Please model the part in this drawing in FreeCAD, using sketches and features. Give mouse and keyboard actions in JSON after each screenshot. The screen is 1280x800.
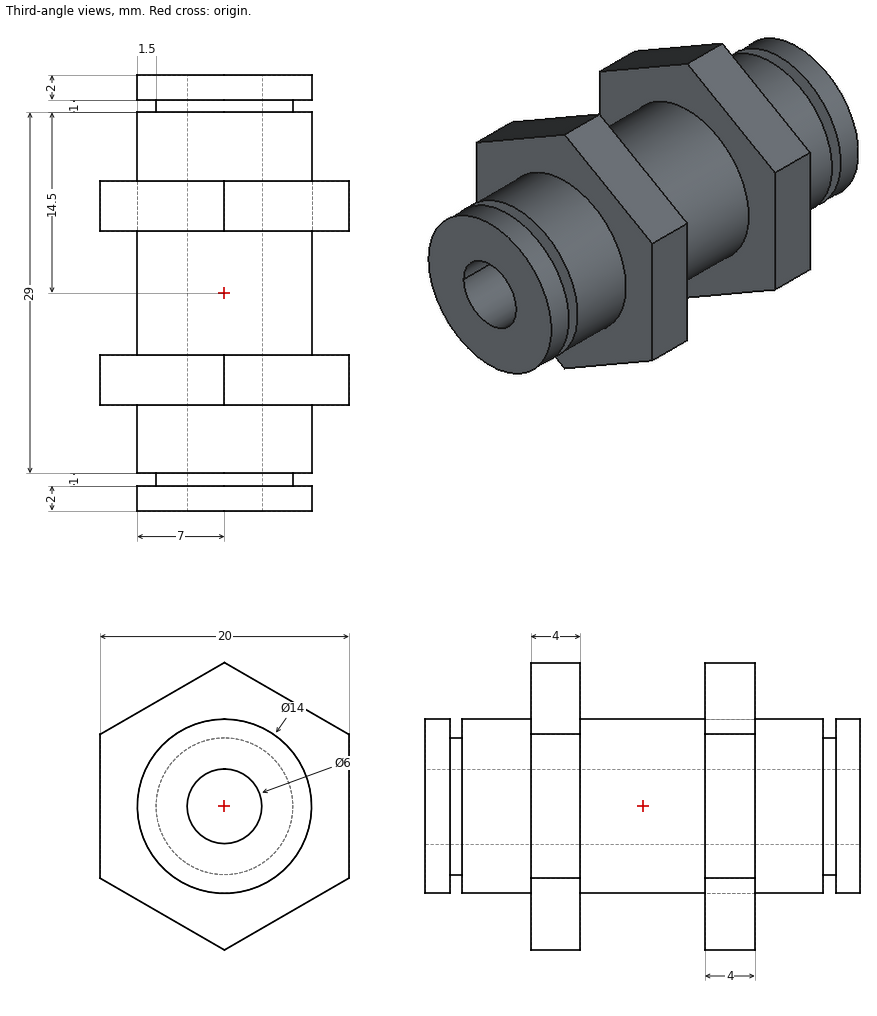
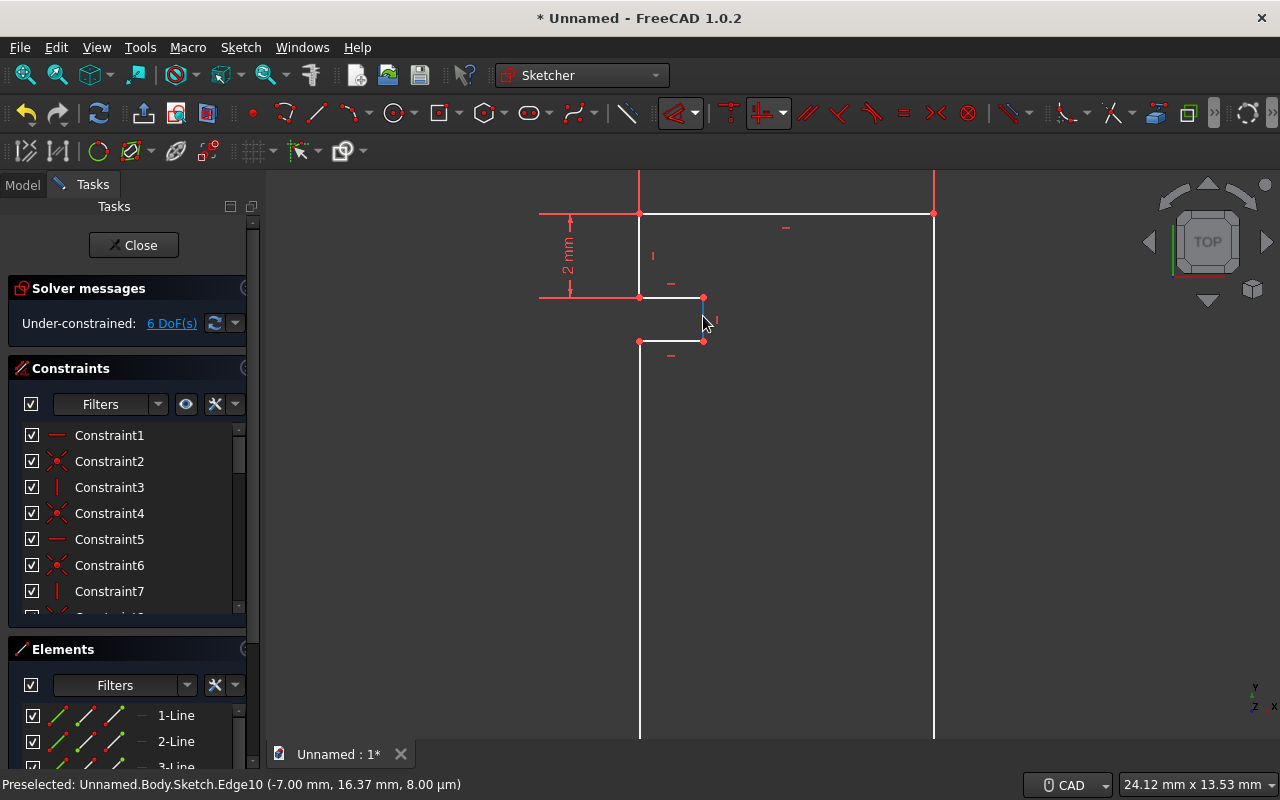
{"action": "left_click", "coordinate": [703, 315]}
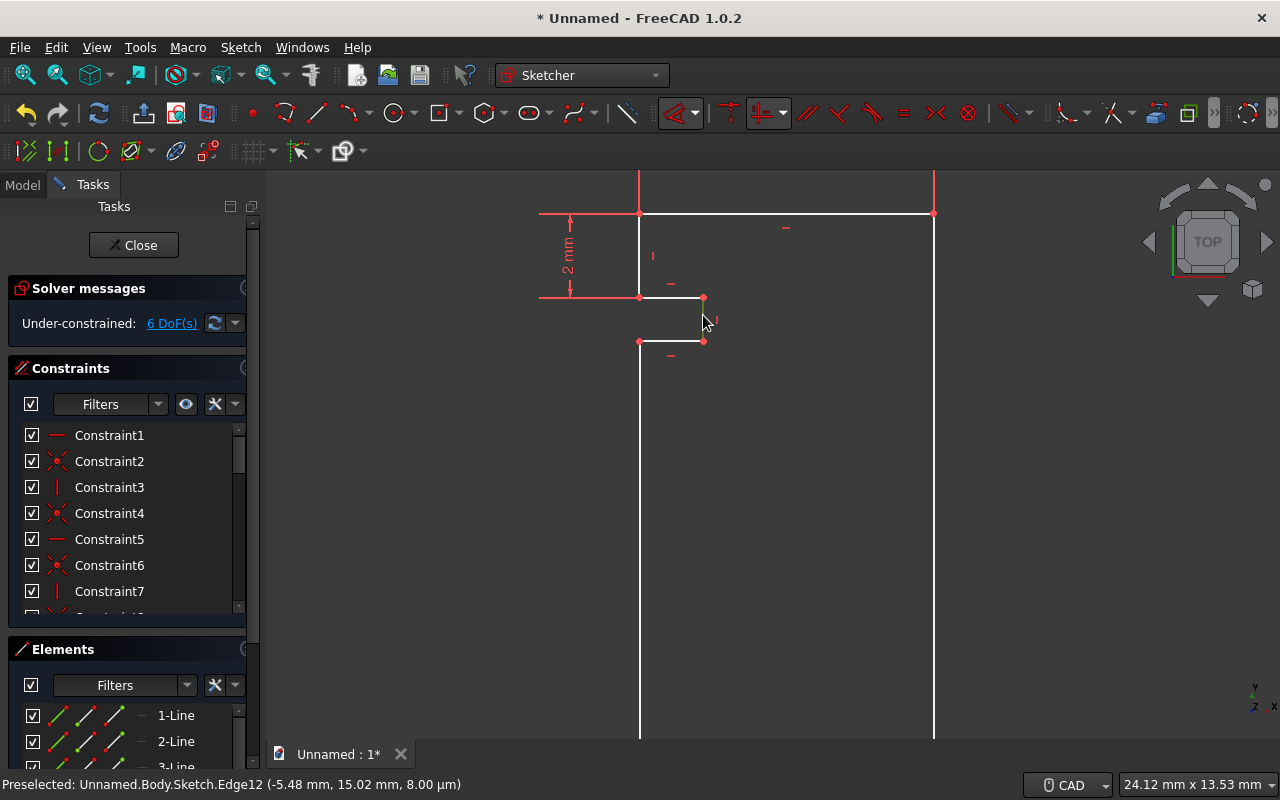
{"action": "left_click", "coordinate": [698, 114]}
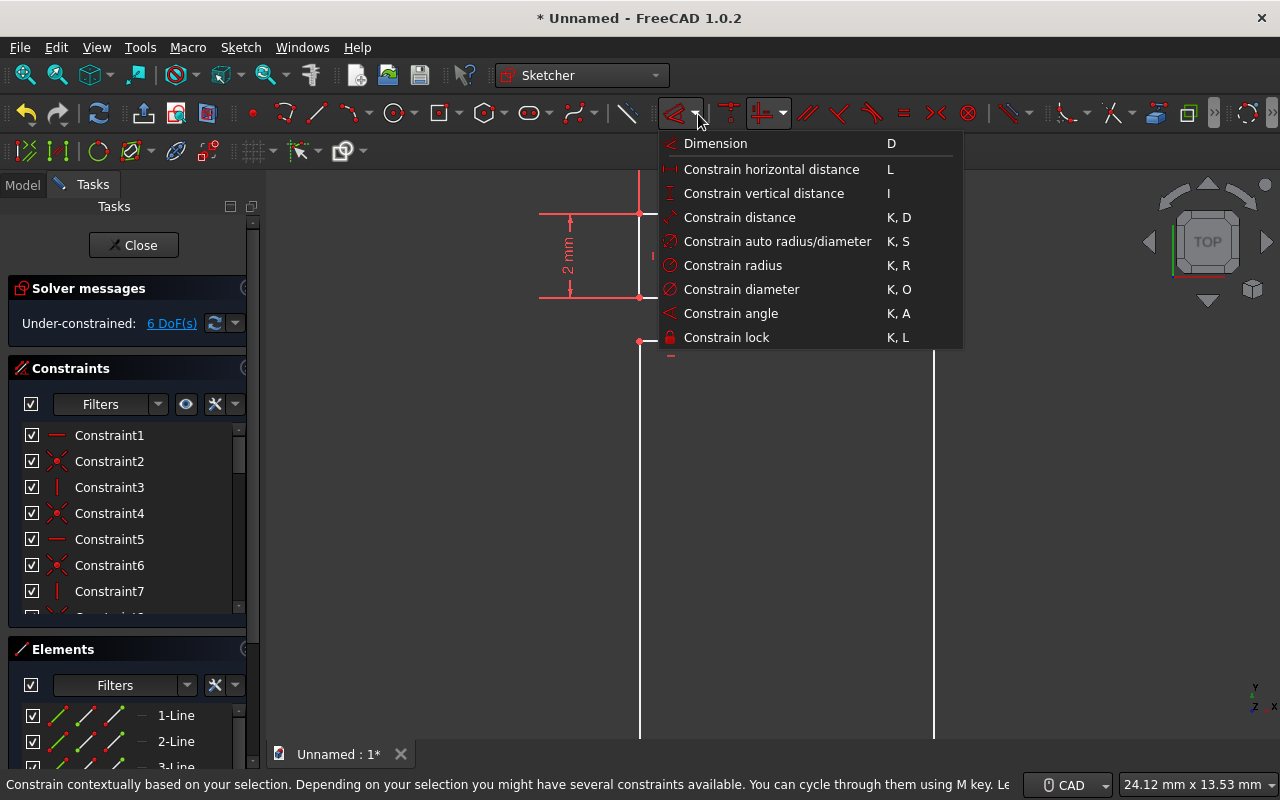
{"action": "left_click", "coordinate": [811, 193]}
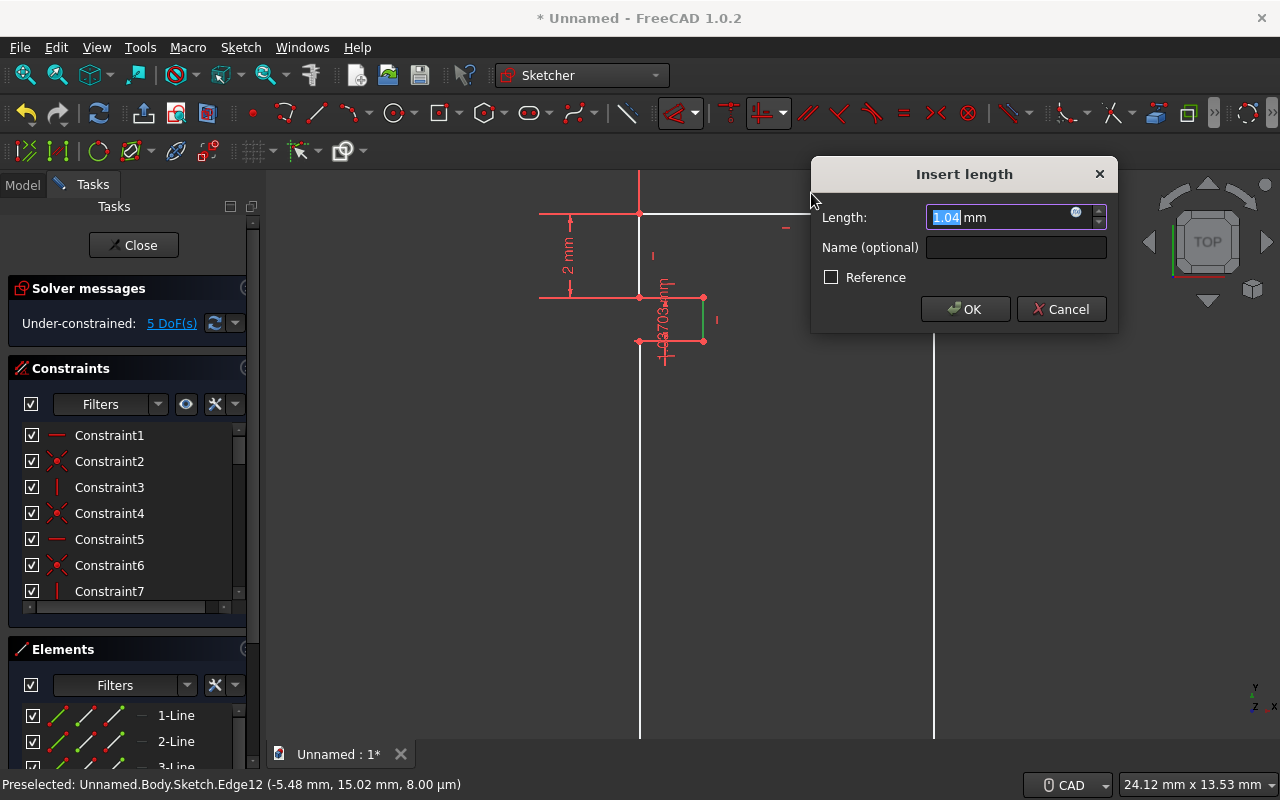
{"action": "type", "text": "1"}
{"action": "key", "text": "Return"}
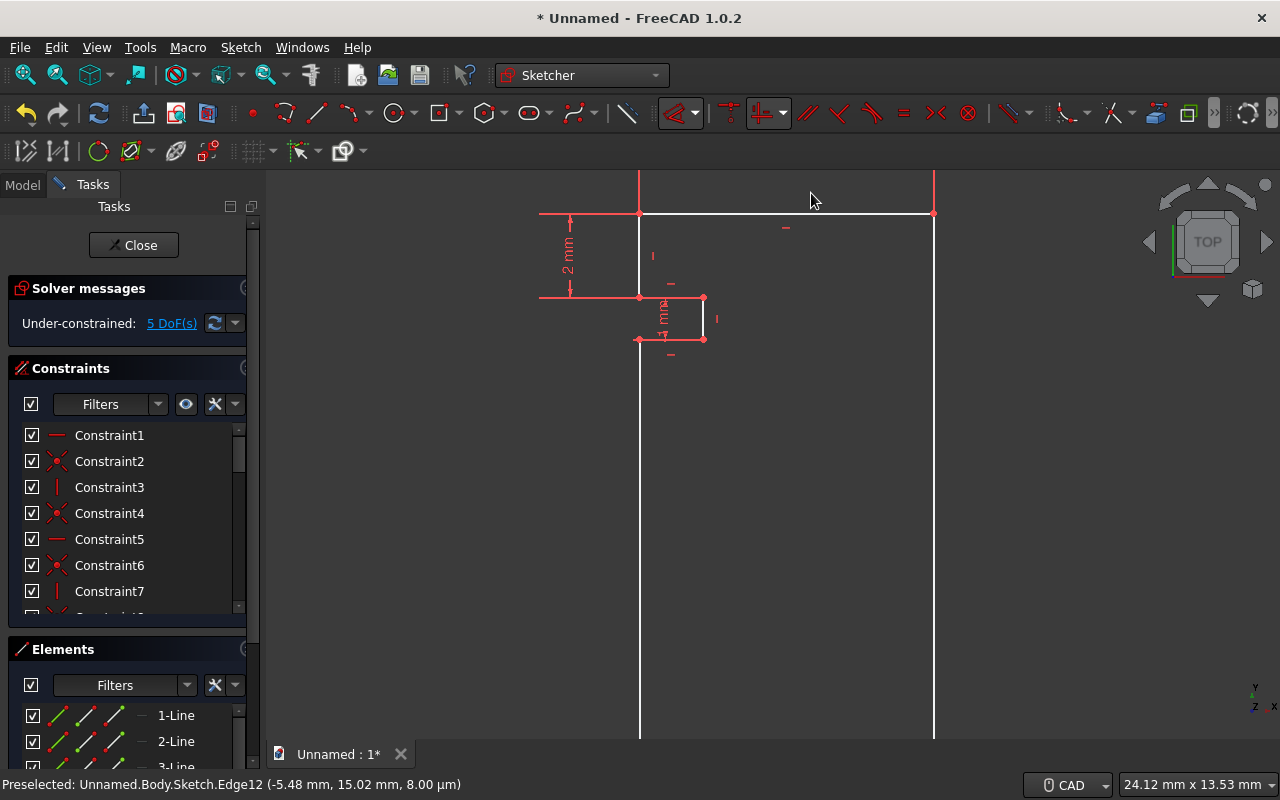
{"action": "scroll", "coordinate": [678, 293], "scroll_direction": "down", "scroll_amount": 7}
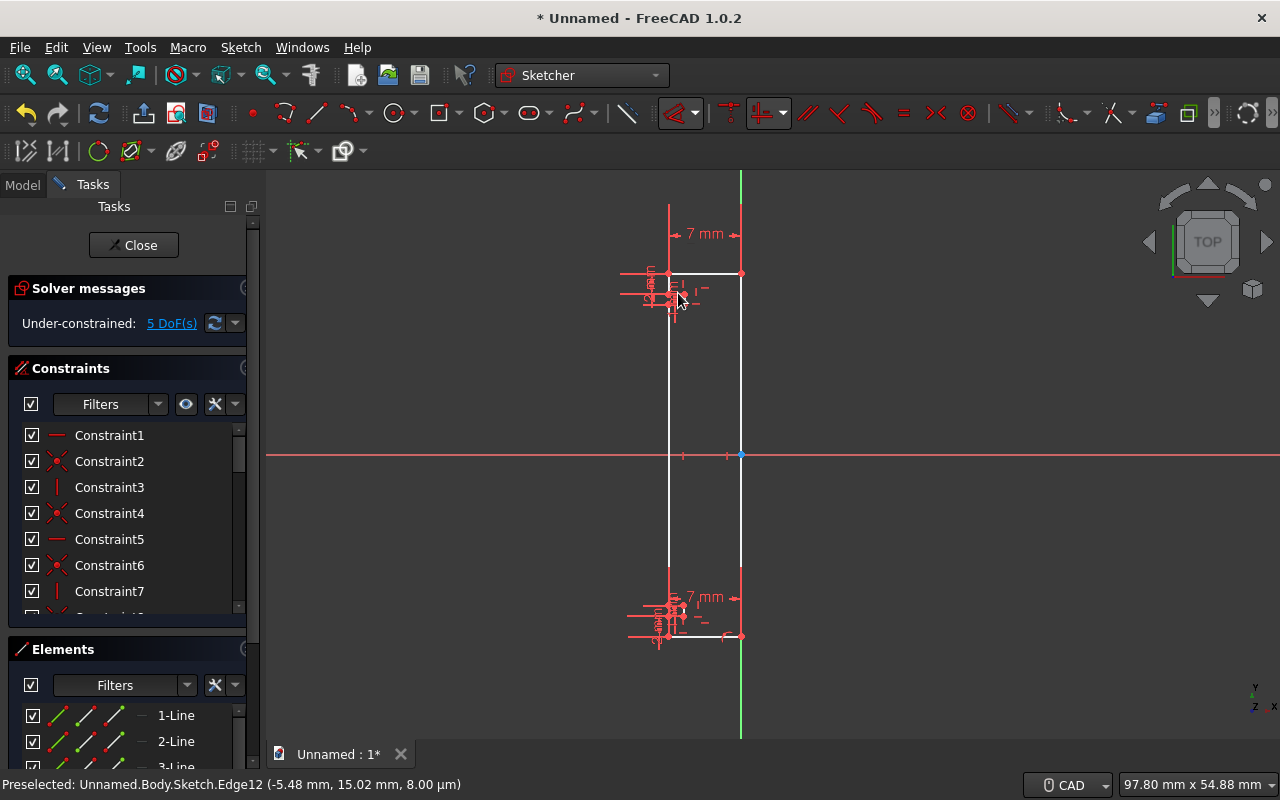
{"action": "left_click", "coordinate": [669, 395]}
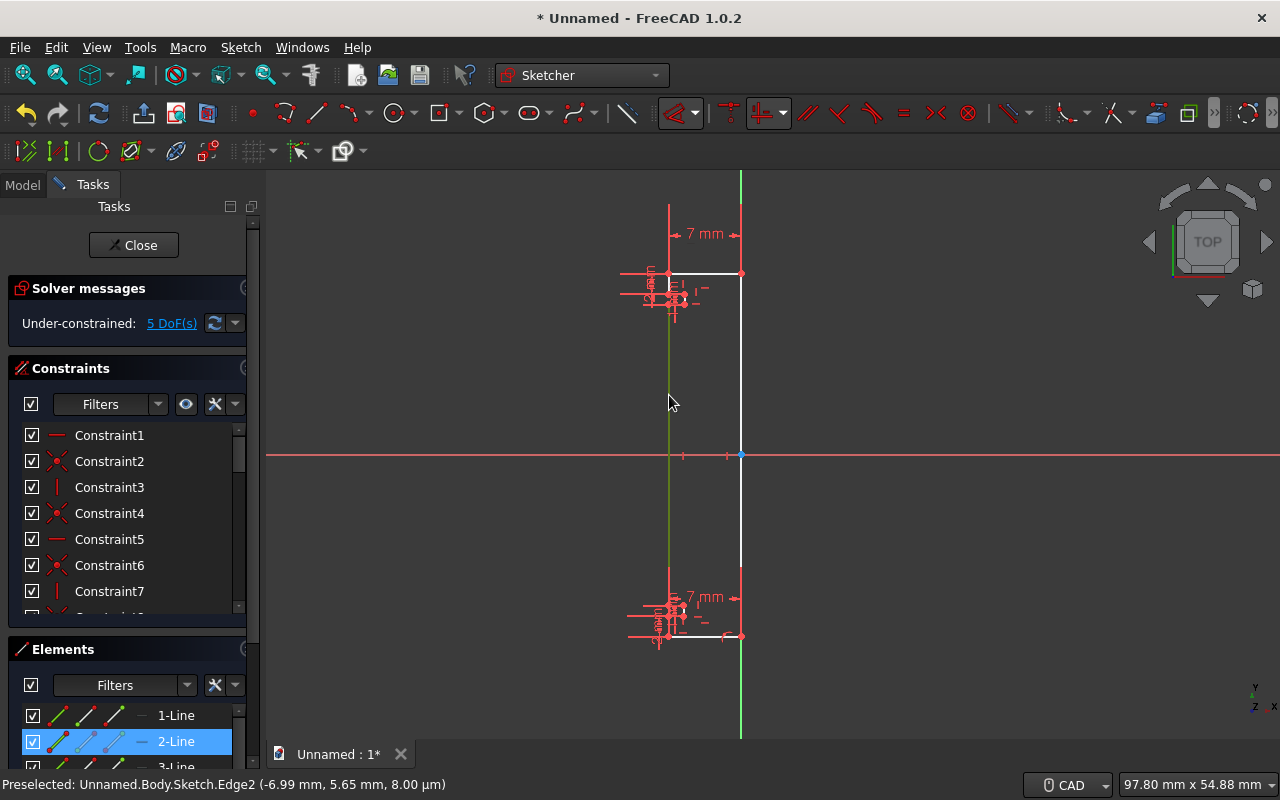
{"action": "key", "text": "i"}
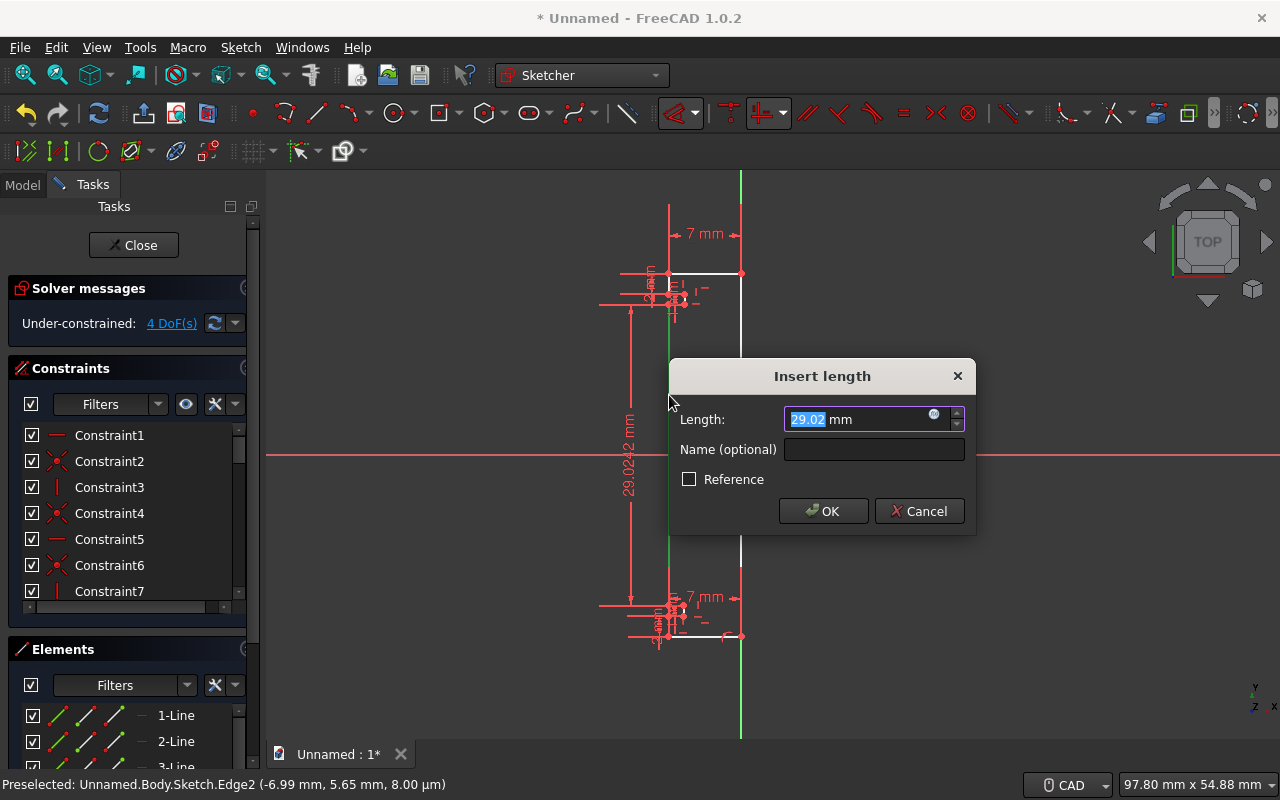
{"action": "type", "text": "29"}
{"action": "key", "text": "Return"}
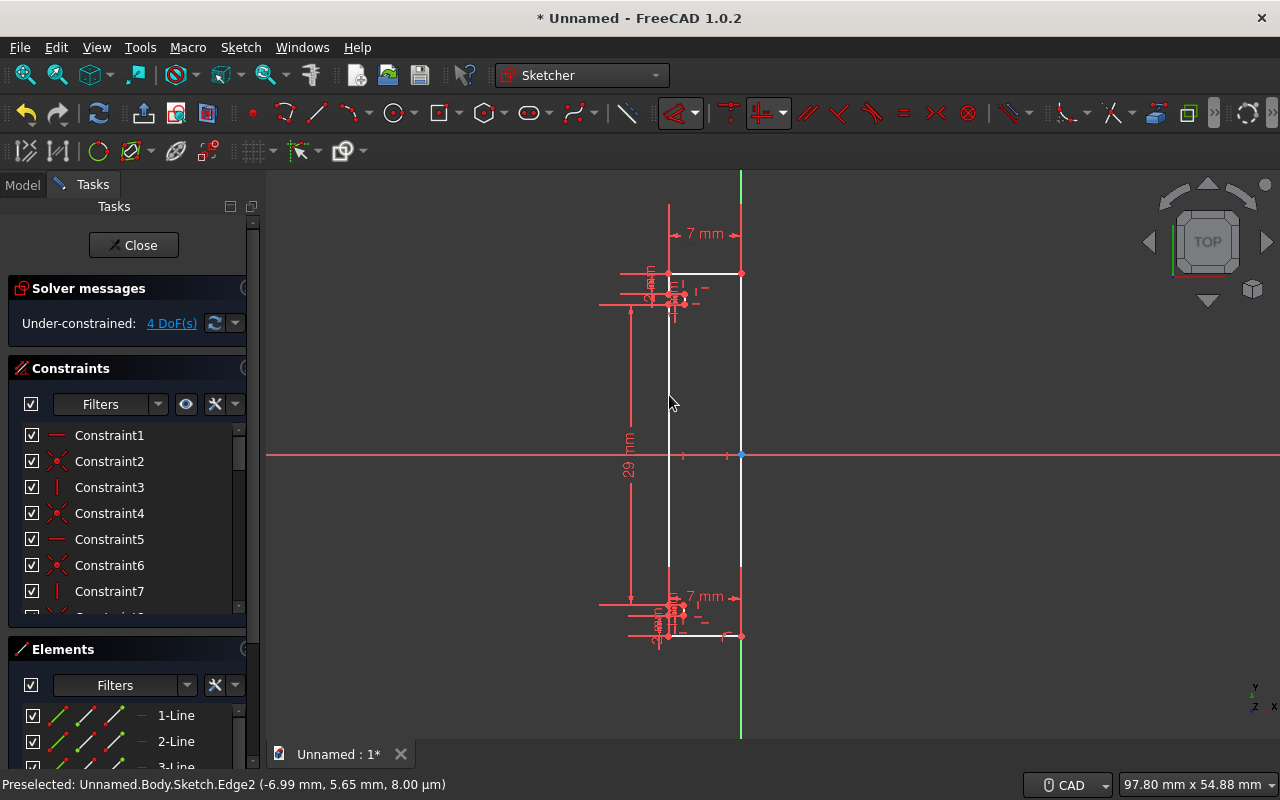
{"action": "left_click", "coordinate": [669, 305]}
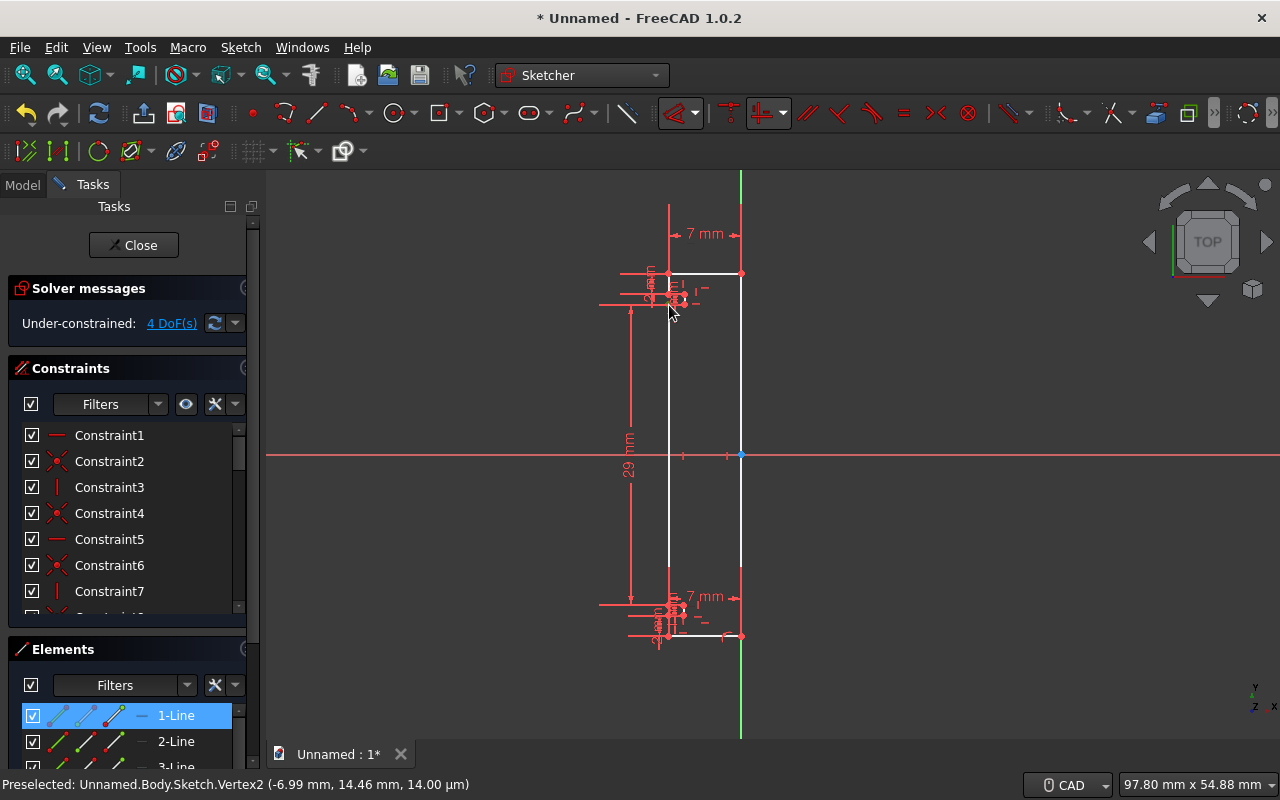
{"action": "key", "text": "l"}